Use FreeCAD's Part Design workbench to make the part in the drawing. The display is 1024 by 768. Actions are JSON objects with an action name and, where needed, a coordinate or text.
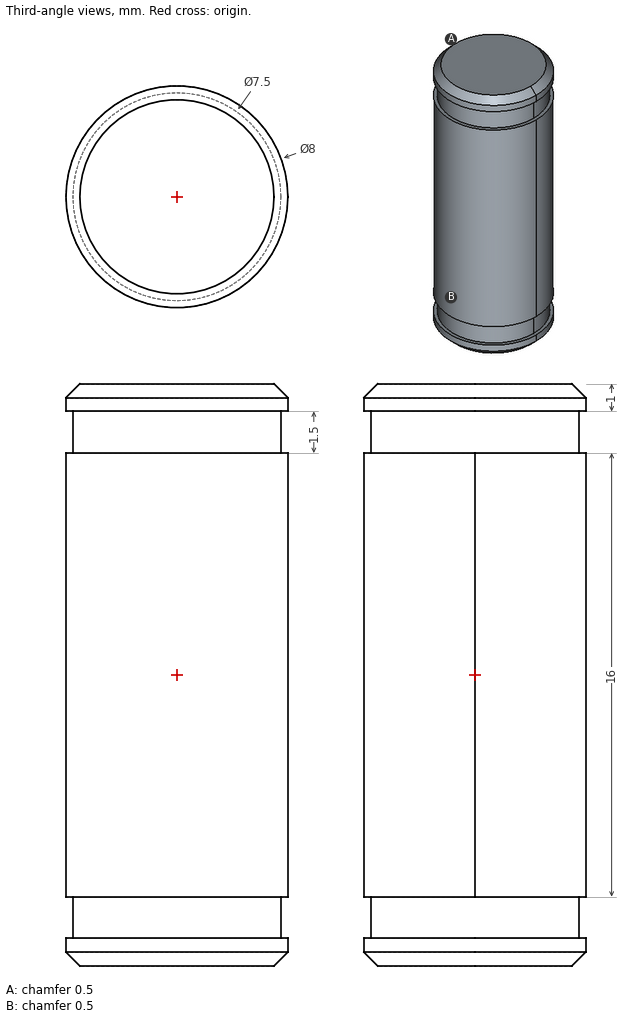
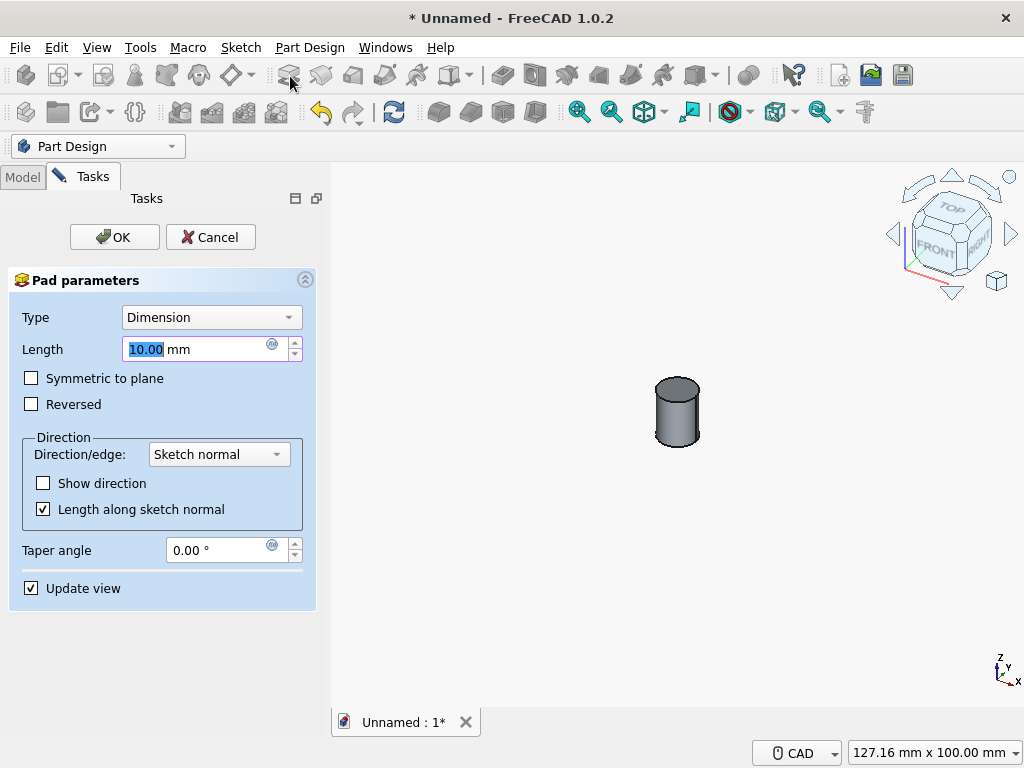
{"action": "type", "text": "16"}
{"action": "key", "text": "Tab"}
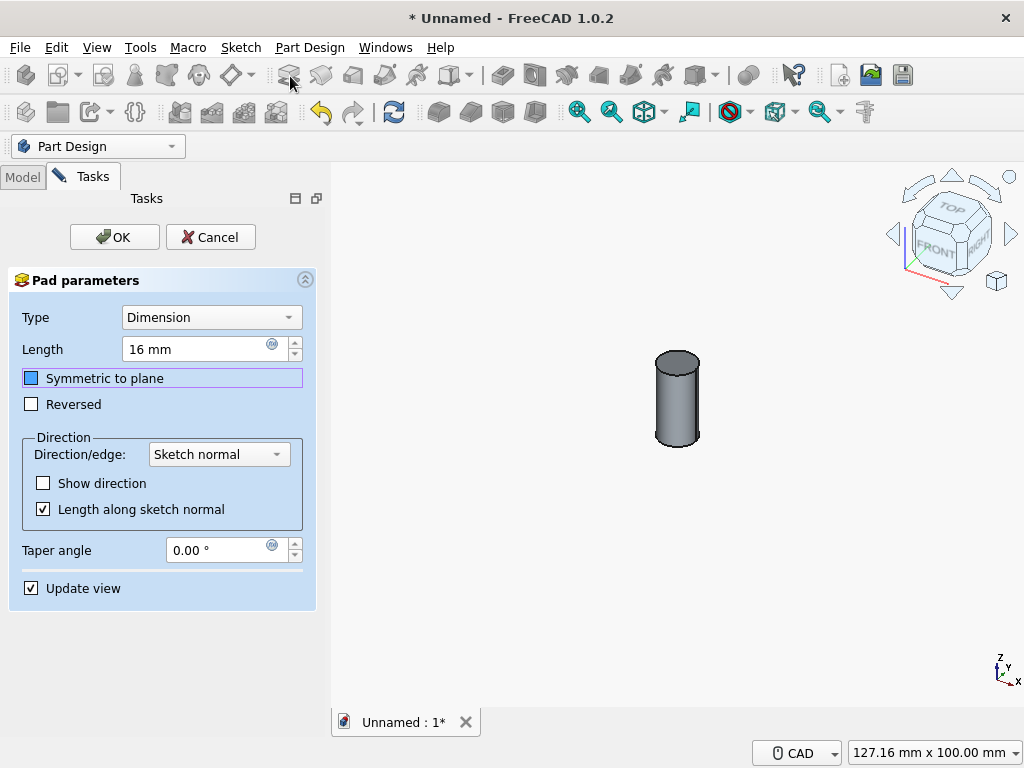
{"action": "left_click", "coordinate": [30, 378]}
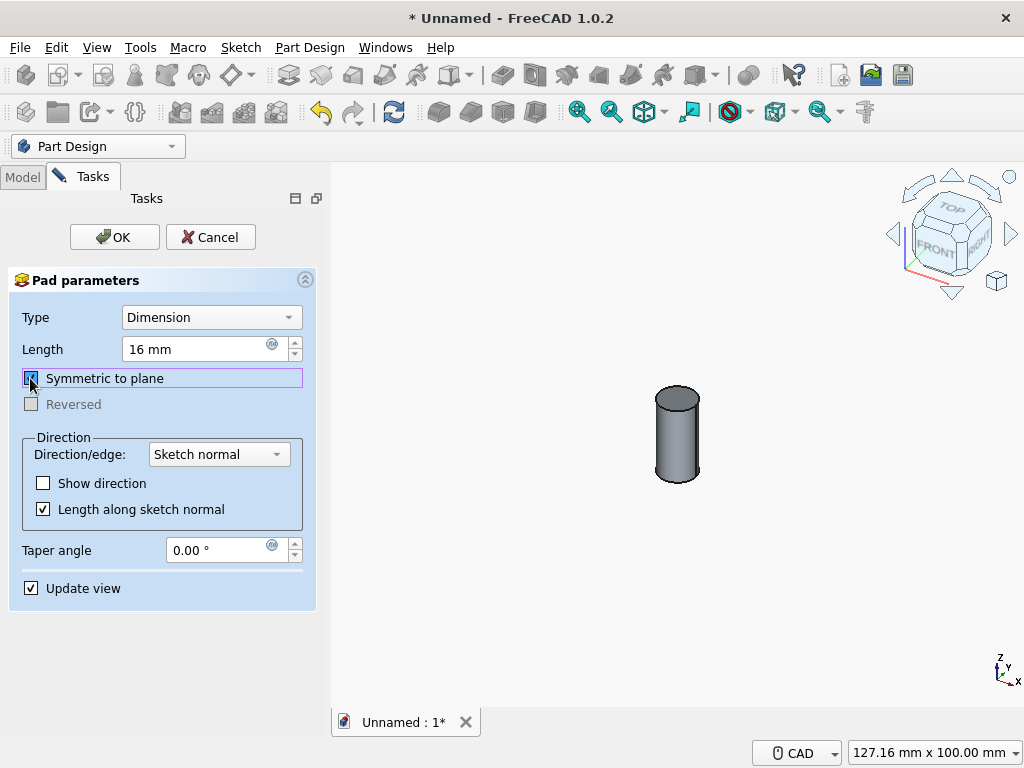
{"action": "left_click", "coordinate": [115, 237]}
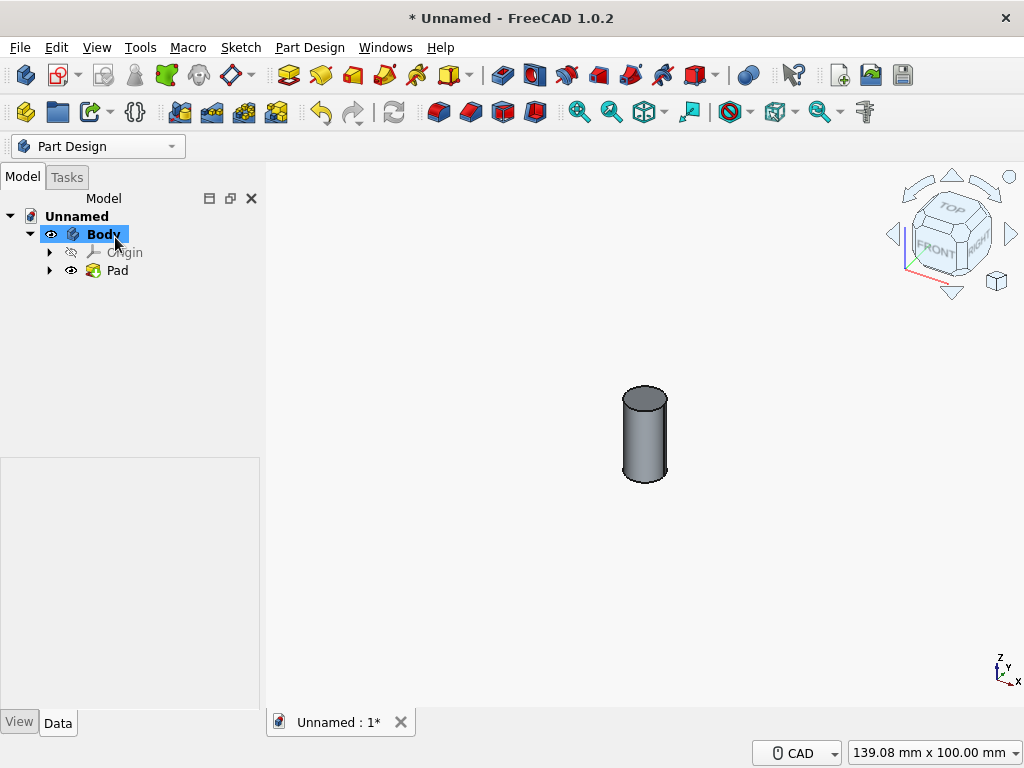
{"action": "key", "text": "v f"}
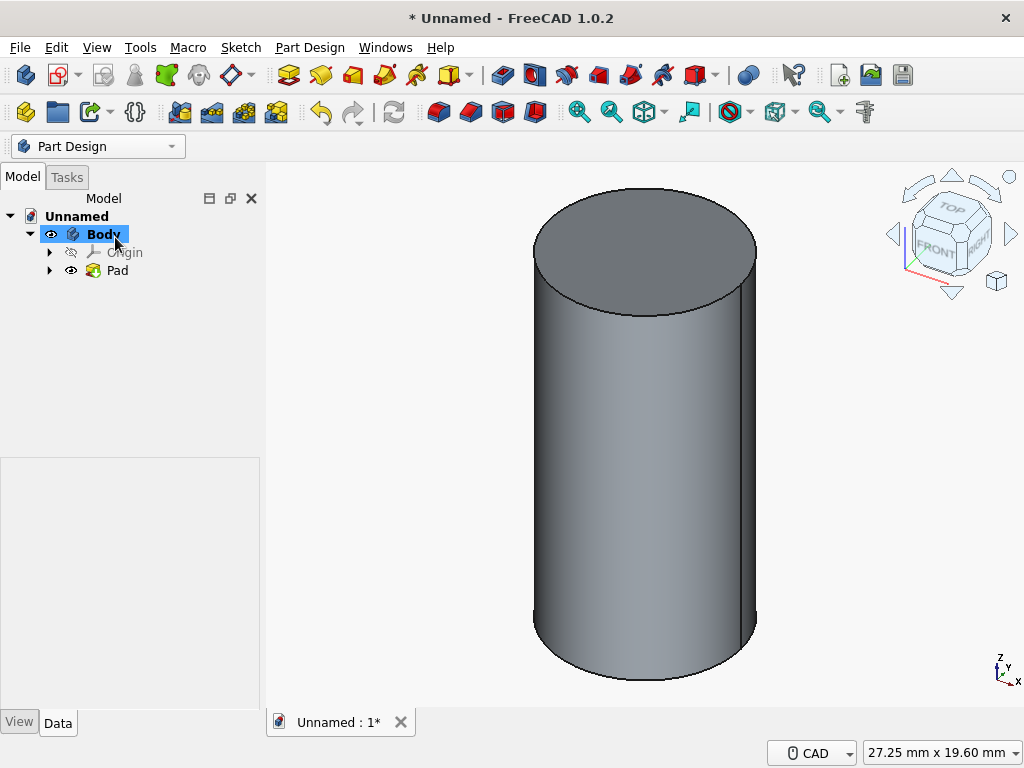
{"action": "left_click", "coordinate": [645, 251]}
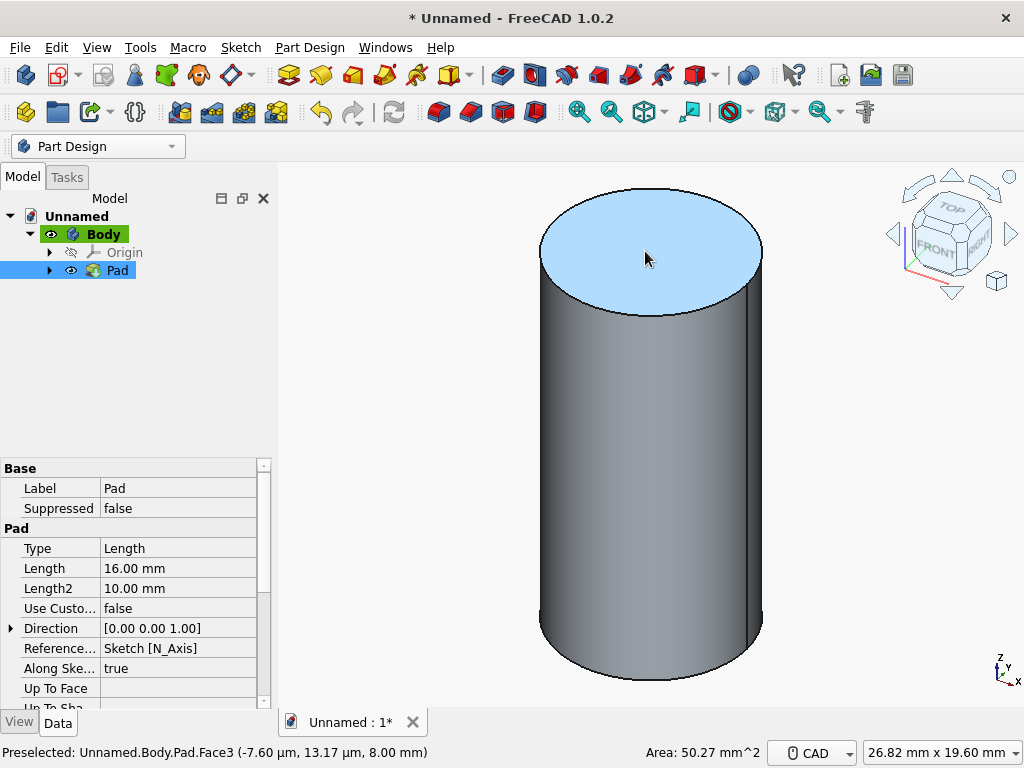
{"action": "left_click", "coordinate": [58, 76]}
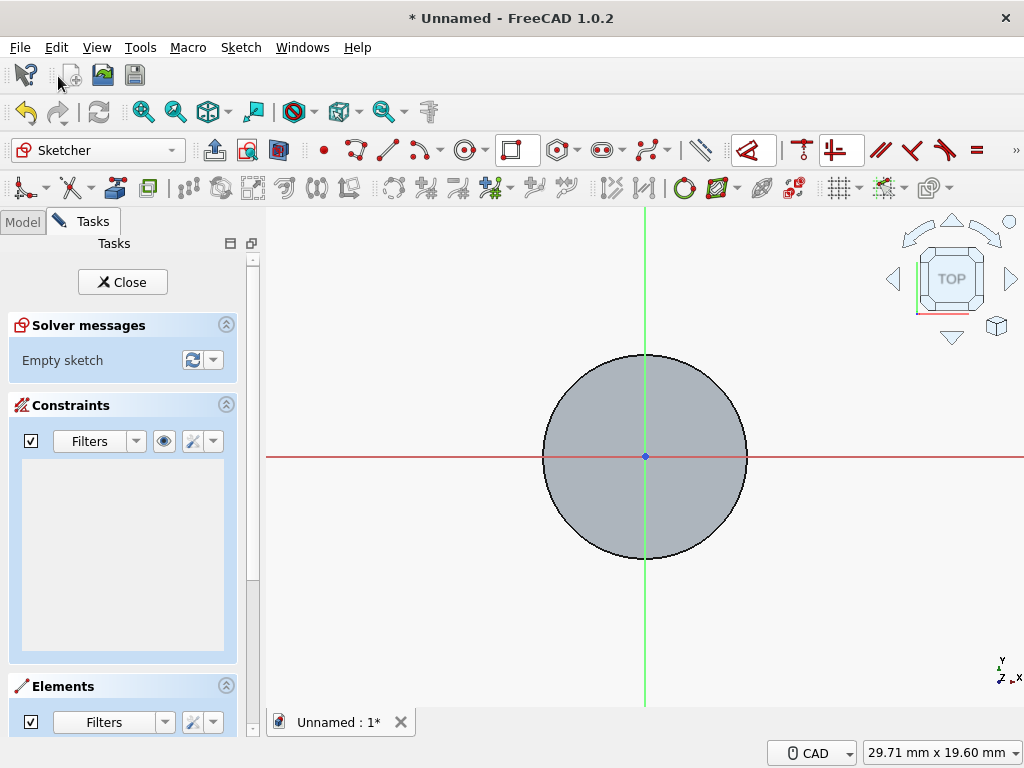
{"action": "scroll", "coordinate": [784, 457], "scroll_direction": "up", "scroll_amount": 2}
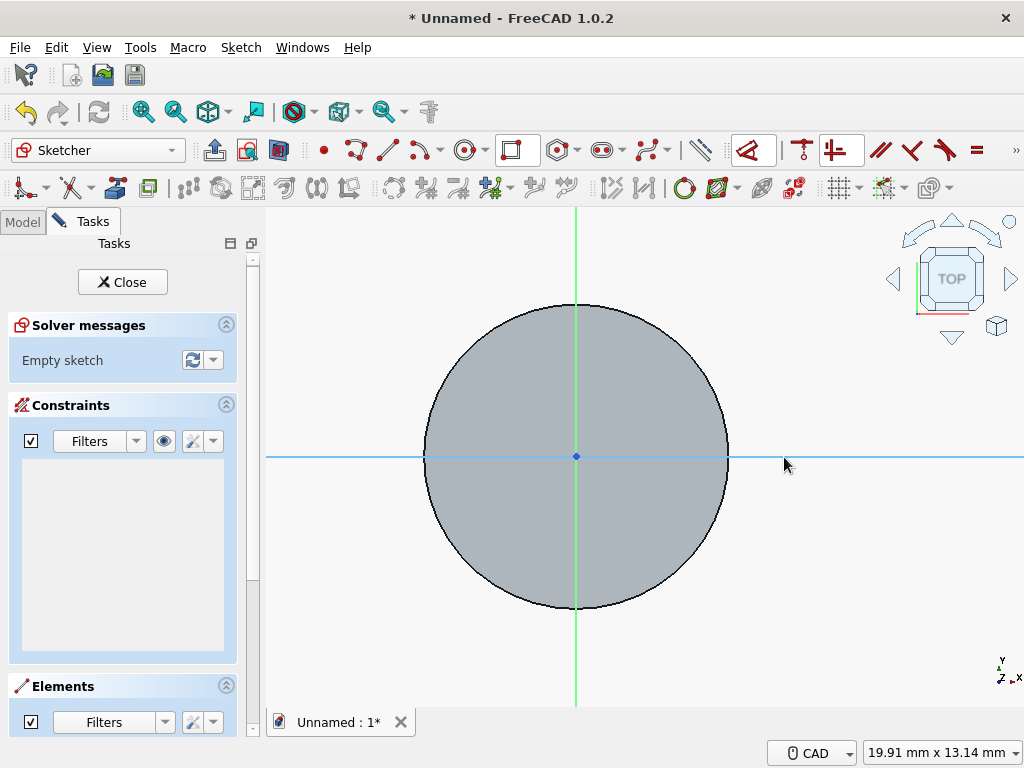
{"action": "key", "text": "g c"}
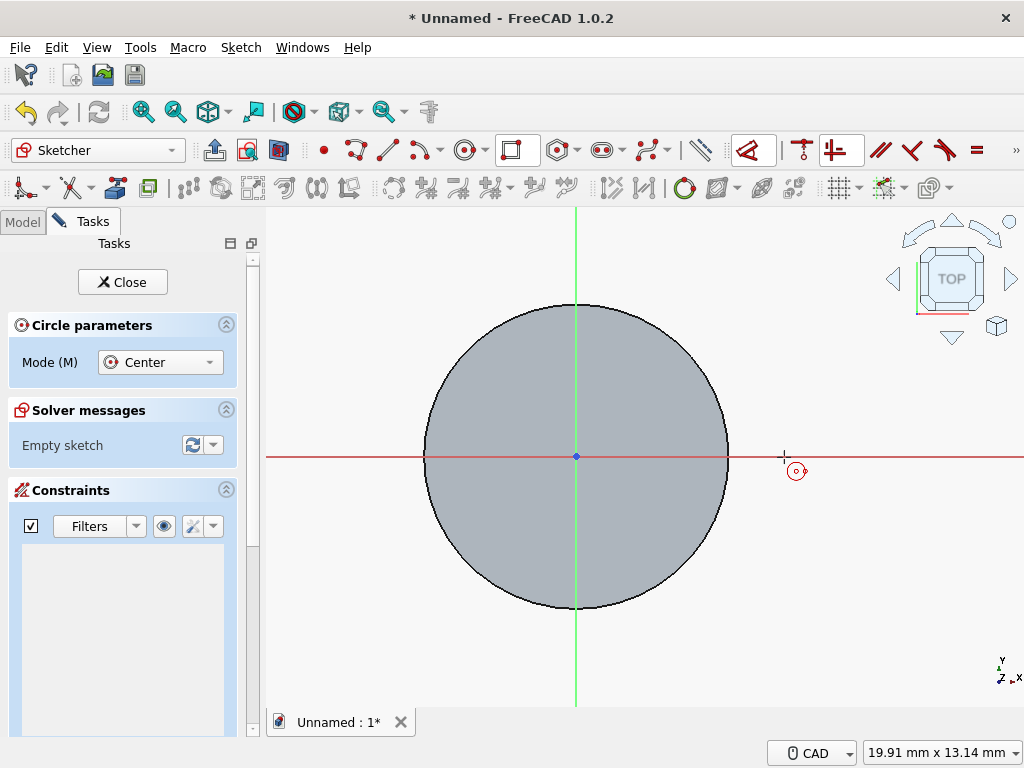
{"action": "left_click", "coordinate": [576, 457]}
{"action": "left_click", "coordinate": [677, 356]}
{"action": "key", "text": "Escape"}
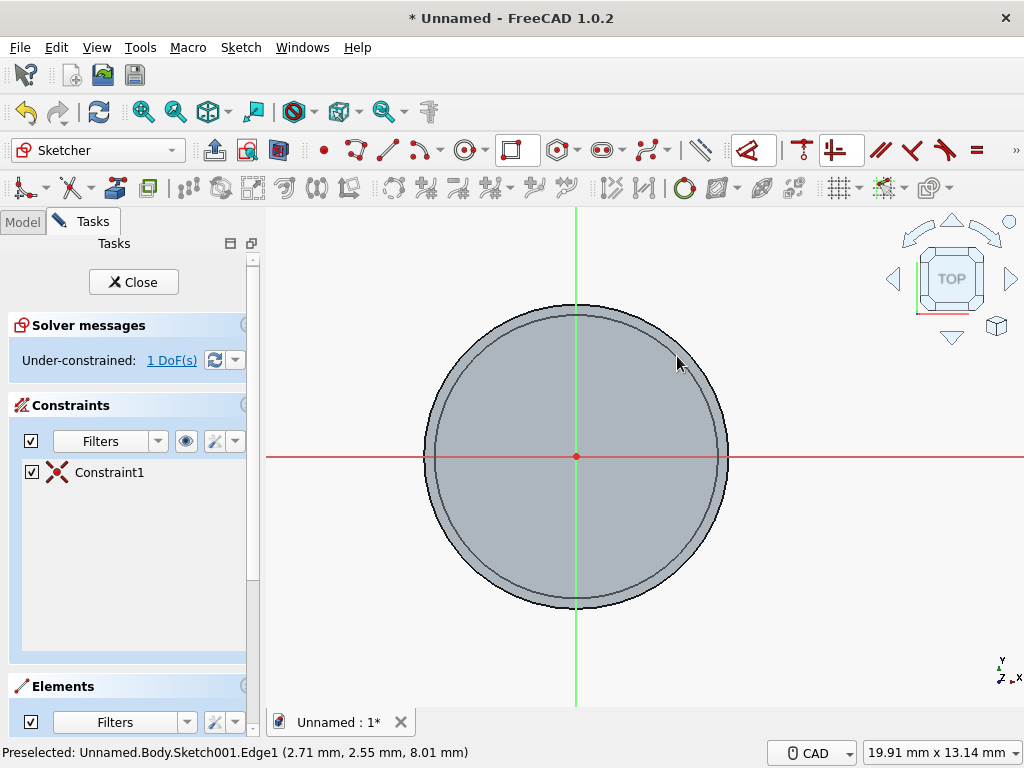
{"action": "left_click", "coordinate": [676, 356]}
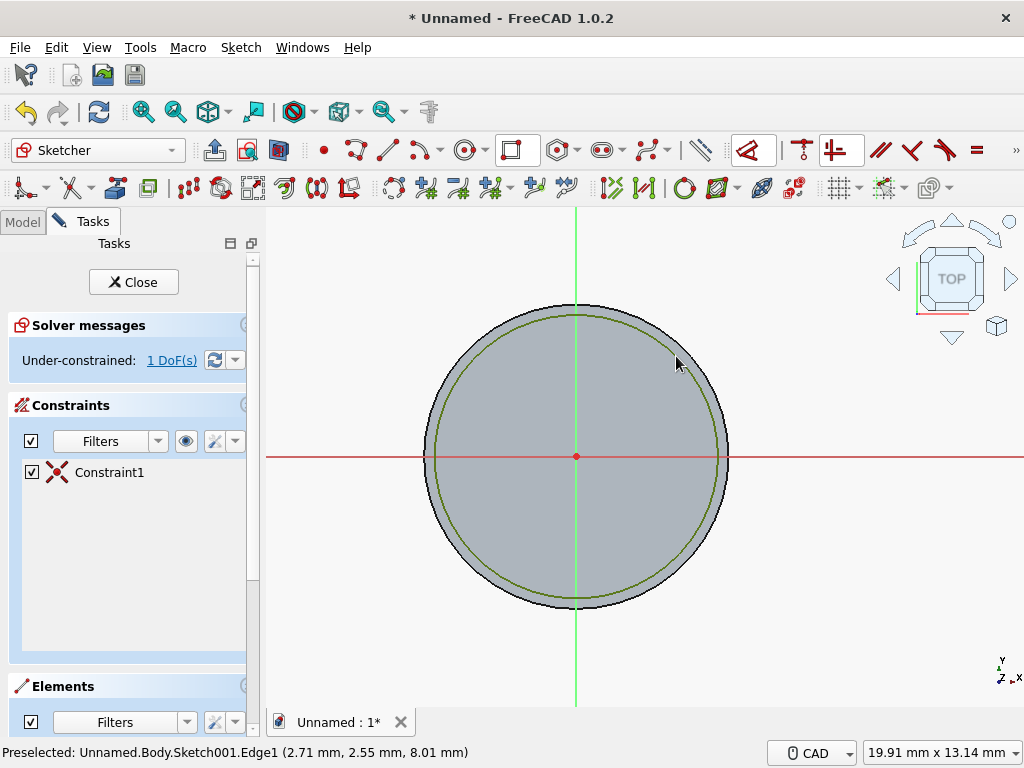
{"action": "key", "text": "k o"}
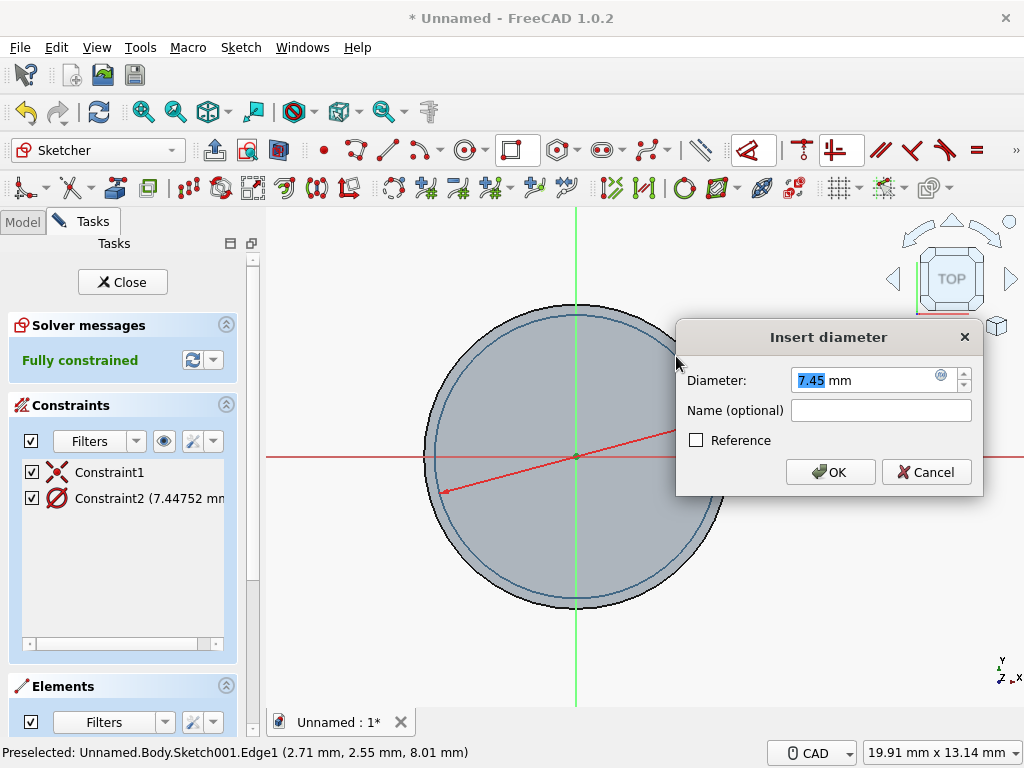
{"action": "type", "text": "7.5"}
{"action": "key", "text": "Return"}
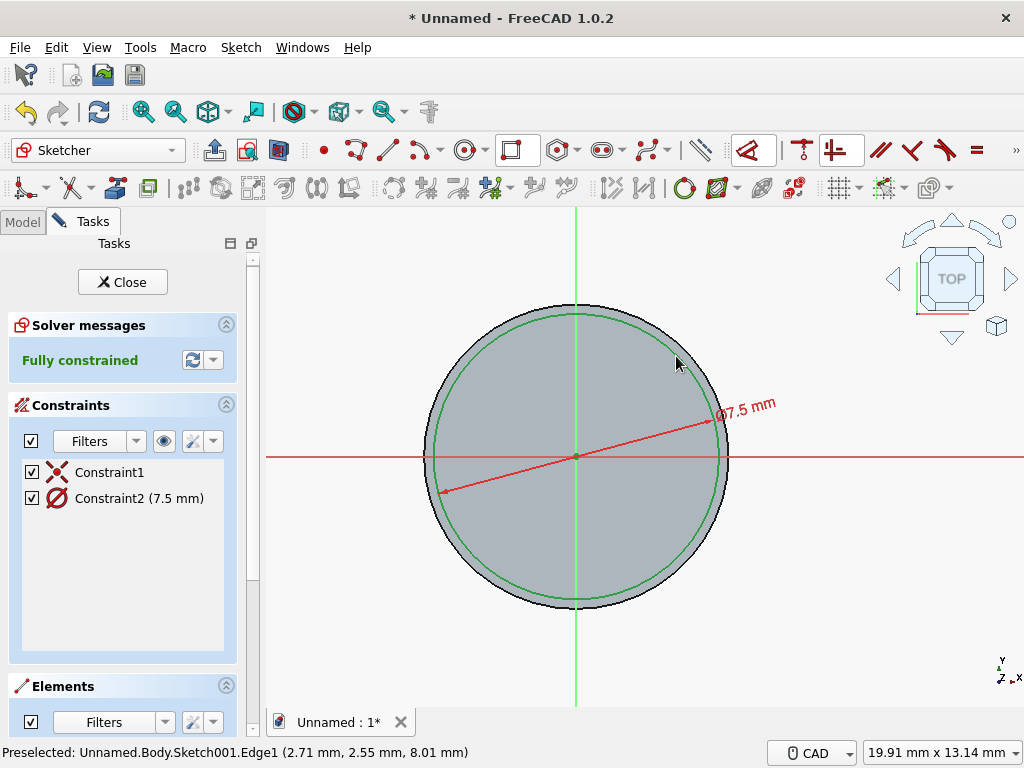
{"action": "left_click", "coordinate": [123, 282]}